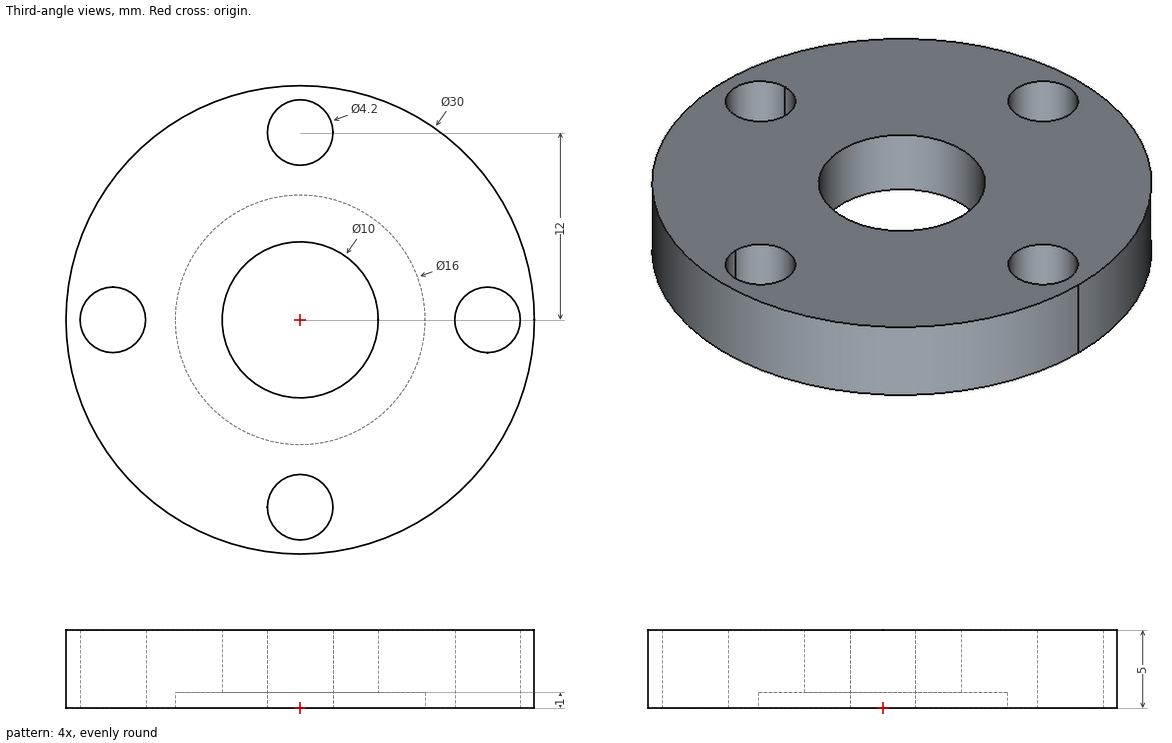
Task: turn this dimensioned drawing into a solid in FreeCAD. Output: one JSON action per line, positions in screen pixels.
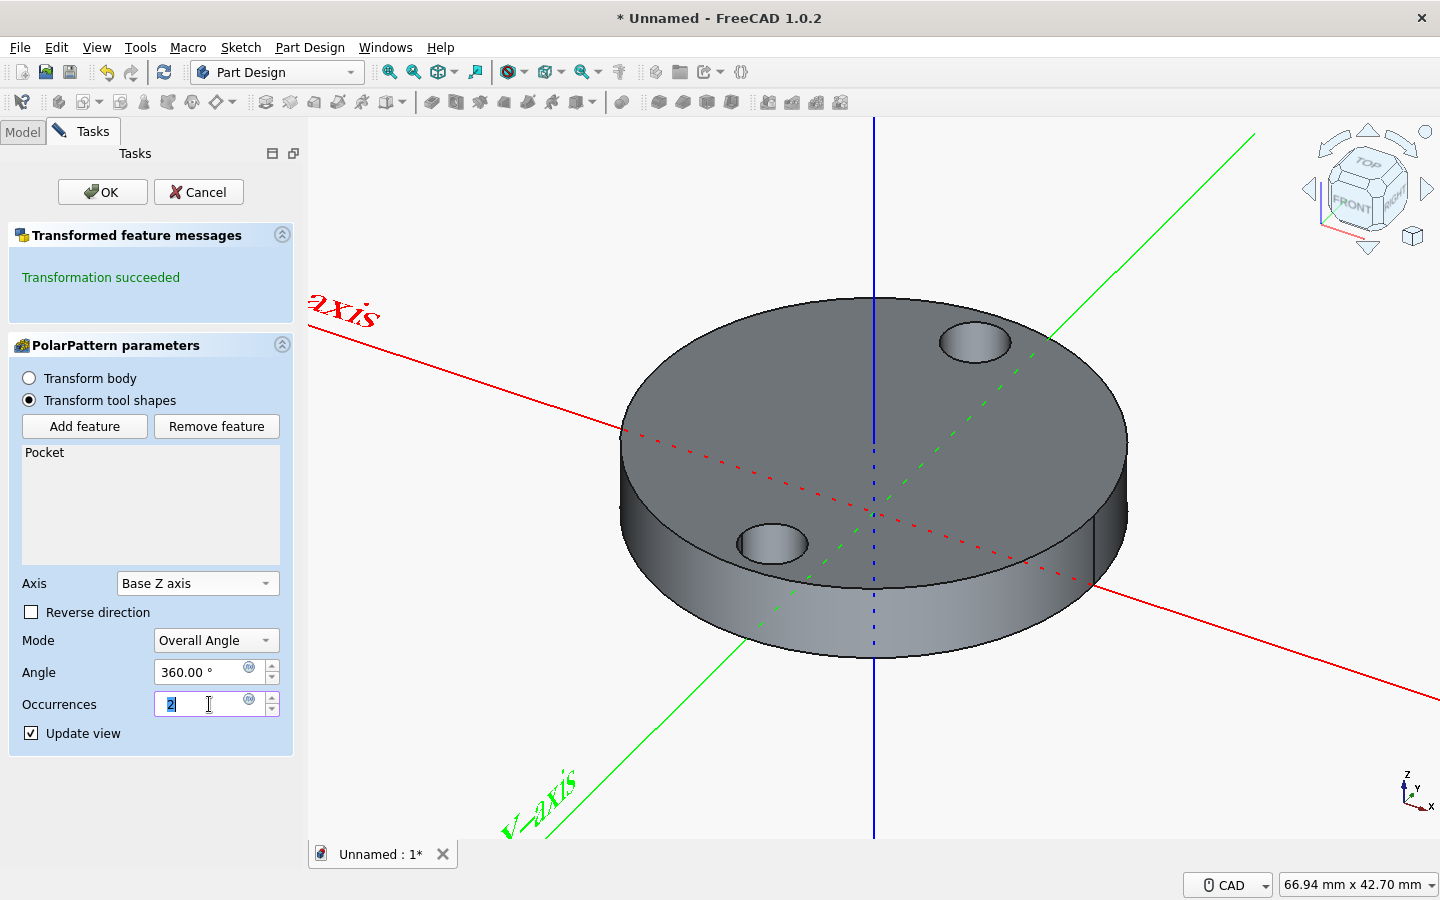
{"action": "type", "text": "4"}
{"action": "key", "text": "Tab"}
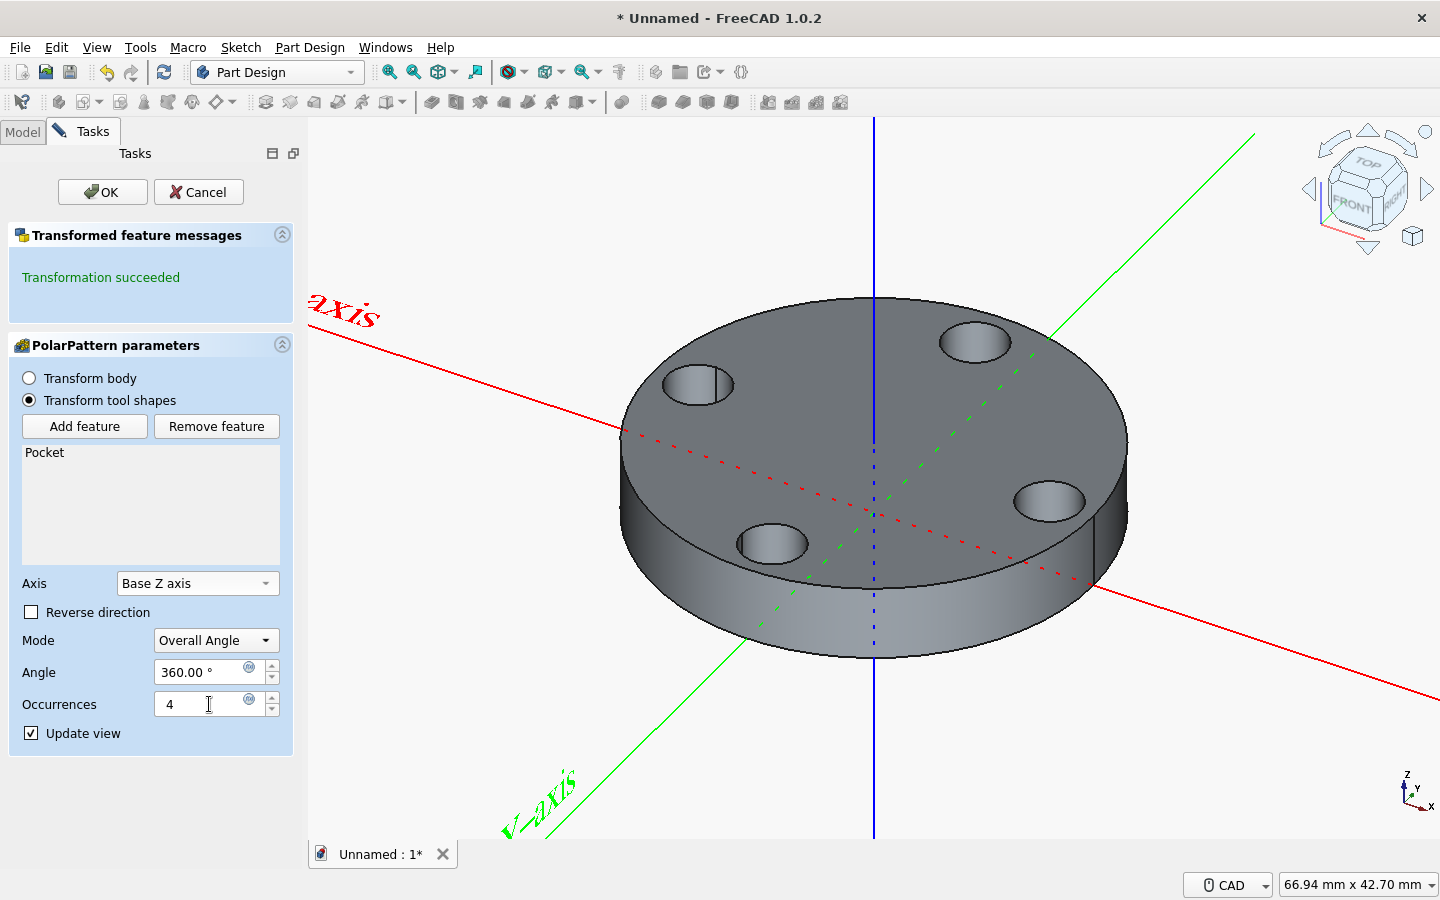
{"action": "left_click", "coordinate": [103, 192]}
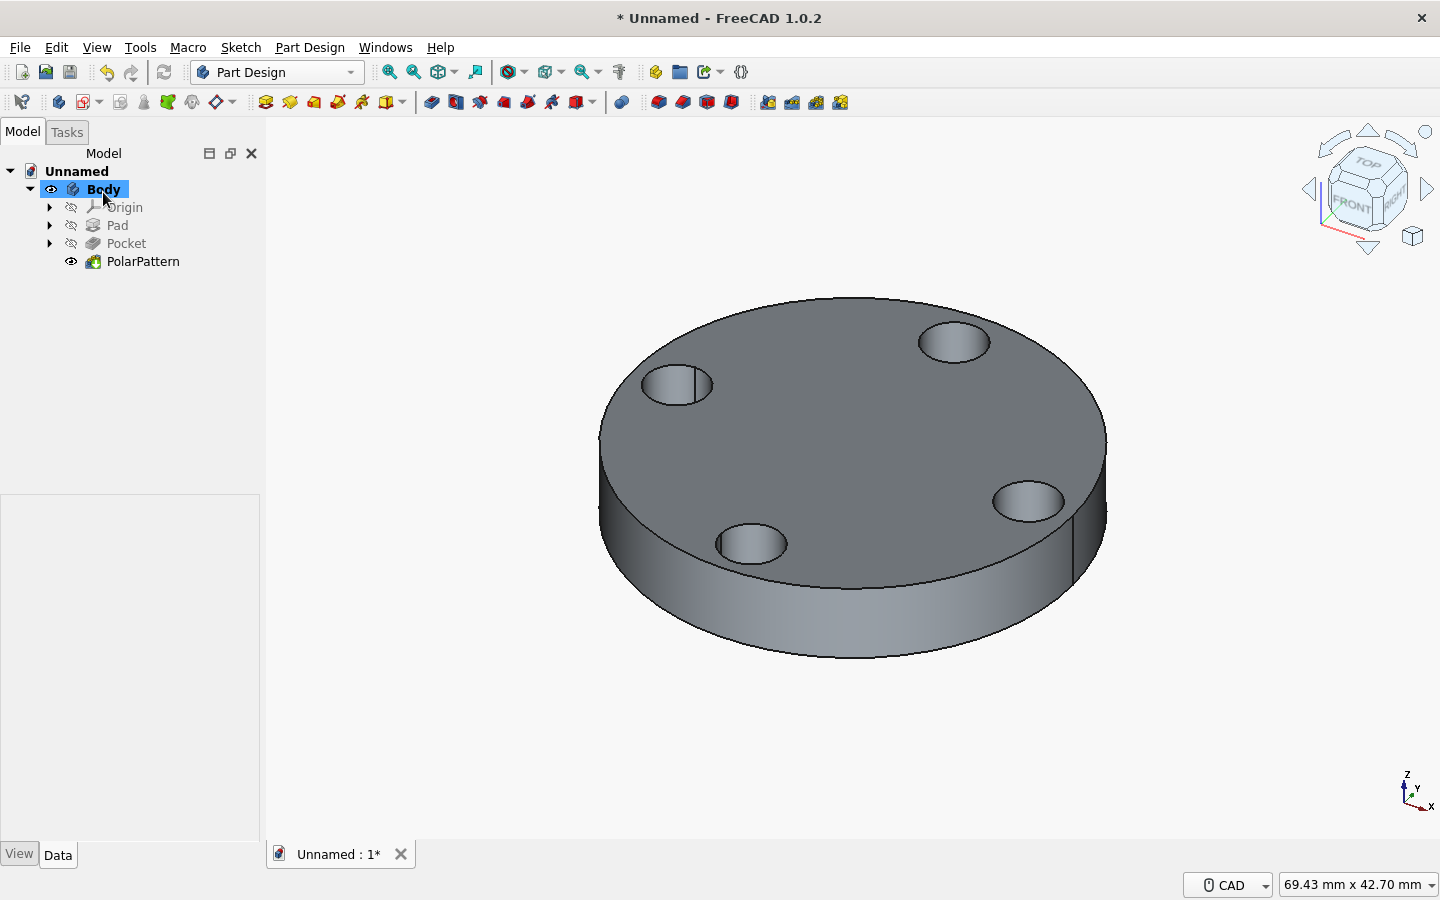
{"action": "key", "text": "5"}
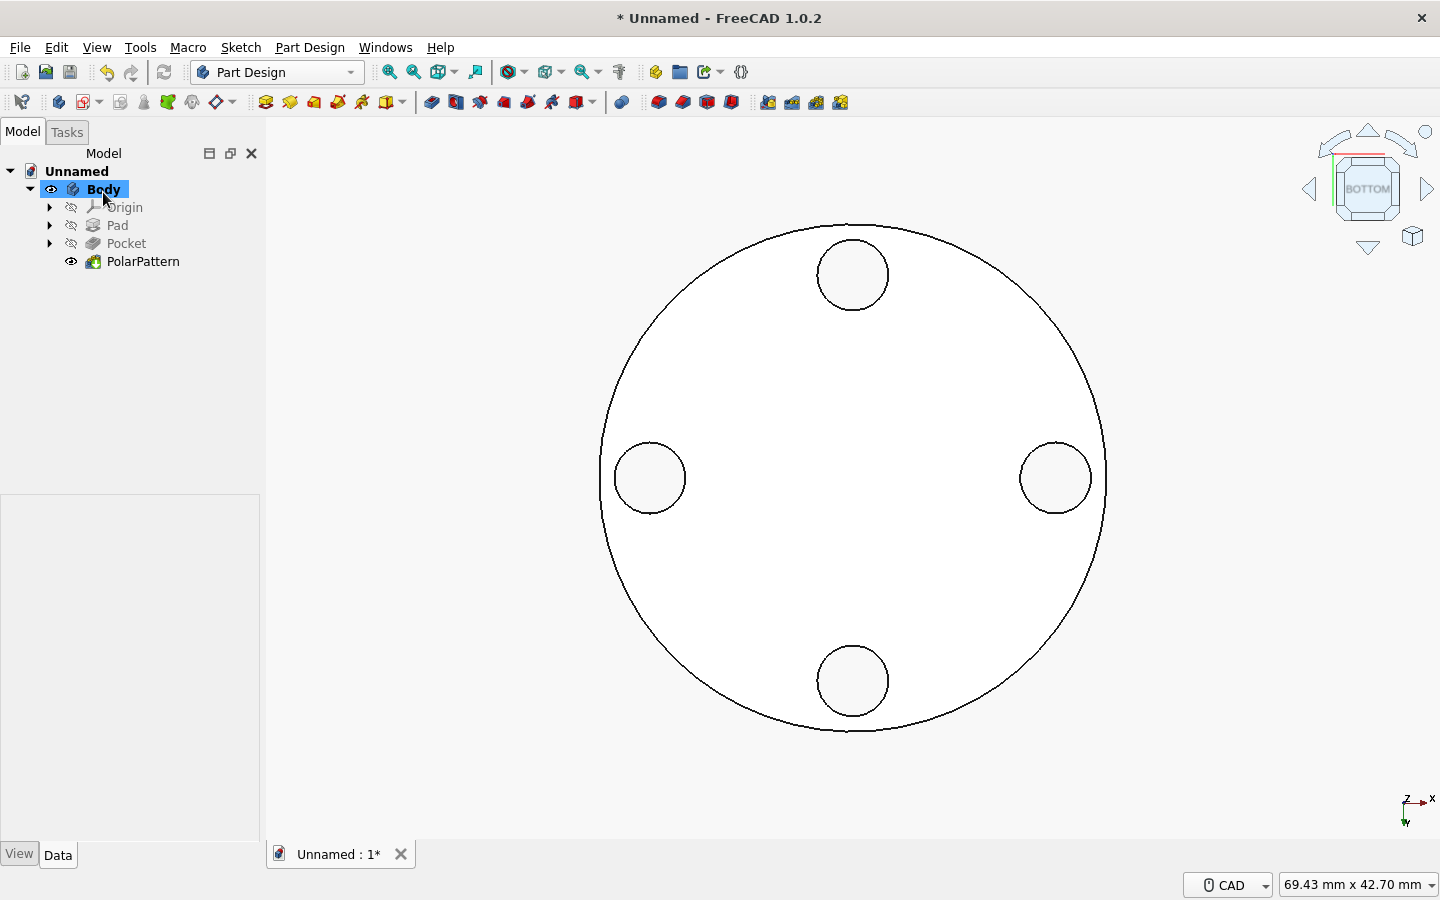
{"action": "left_click", "coordinate": [853, 477]}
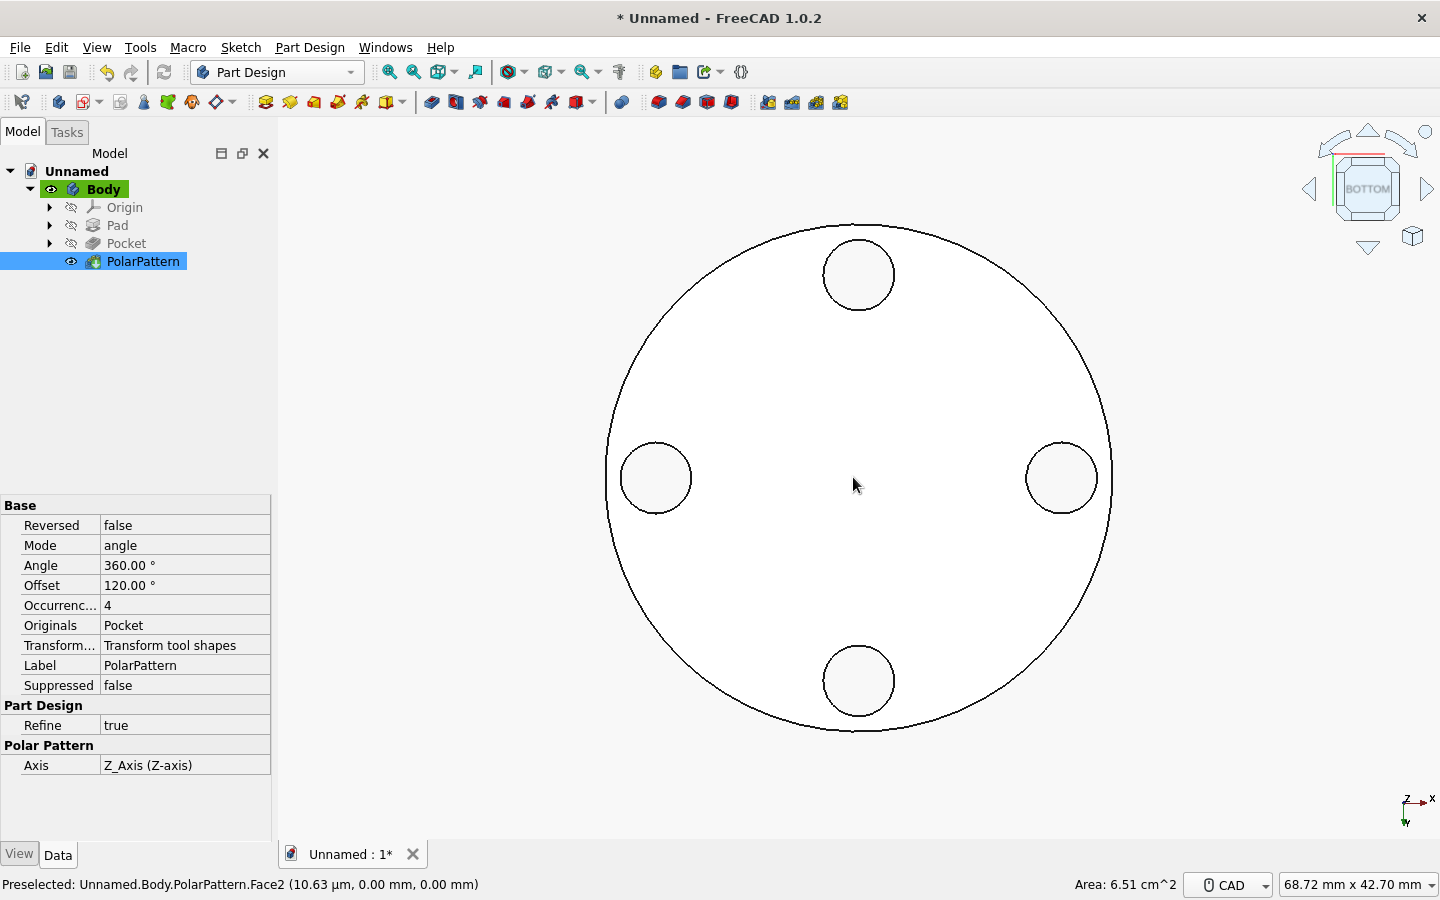
{"action": "left_click", "coordinate": [84, 102]}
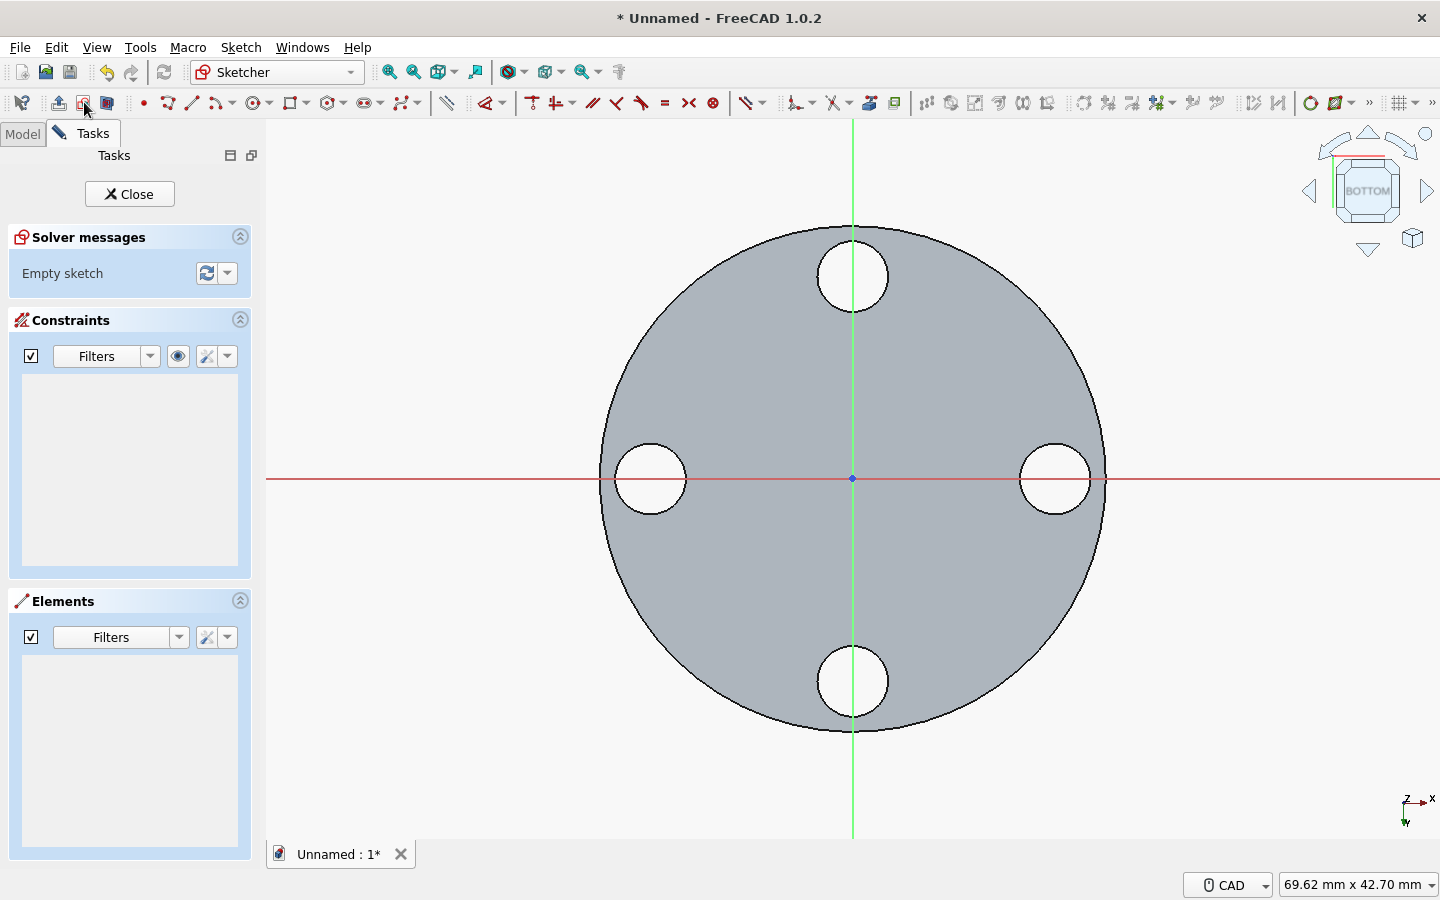
{"action": "scroll", "coordinate": [936, 479], "scroll_direction": "up", "scroll_amount": 3}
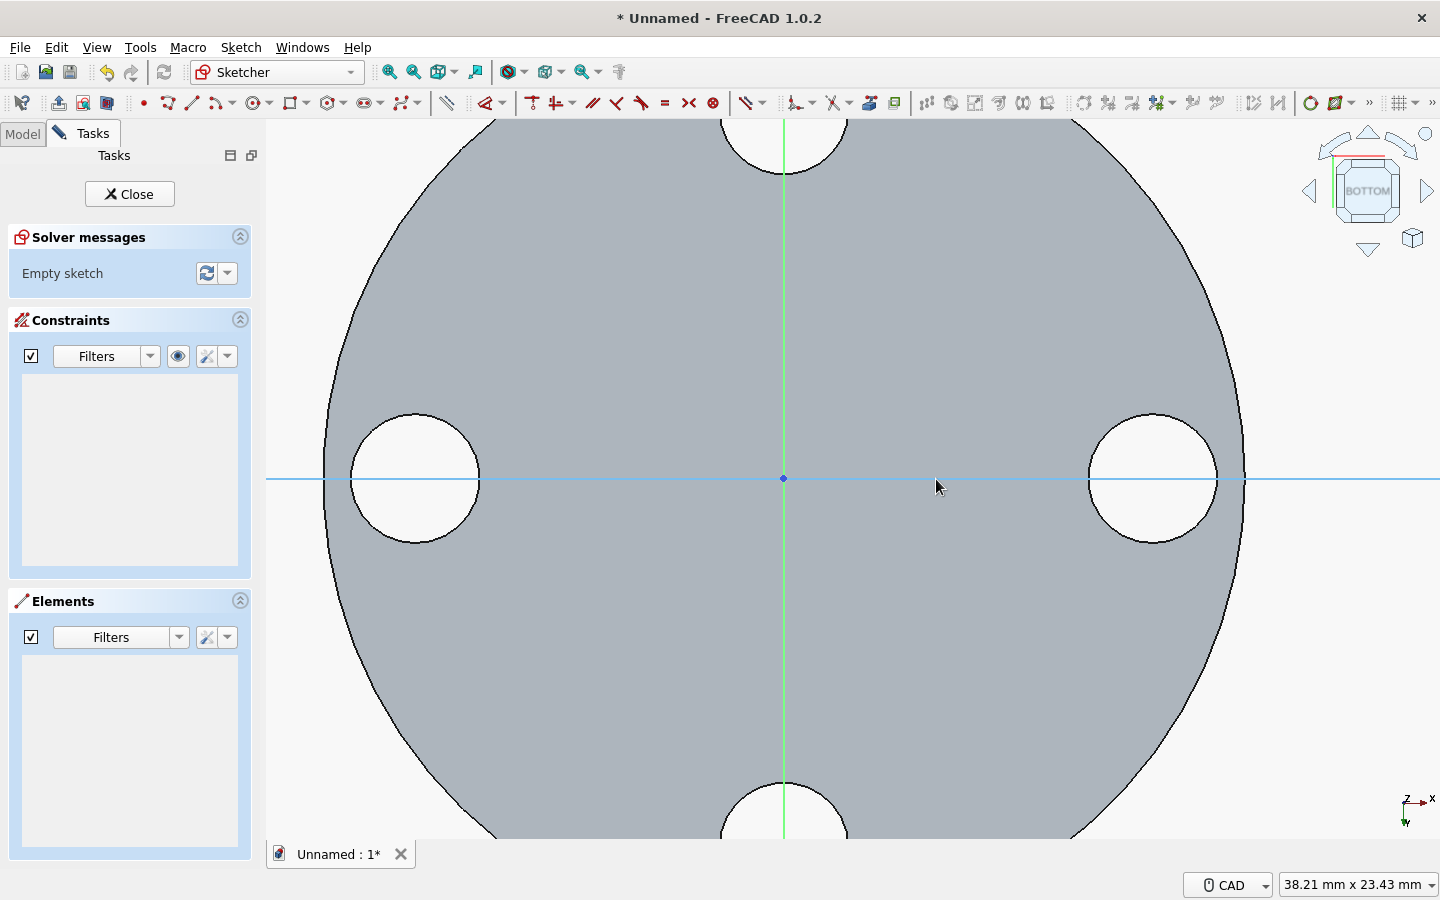
{"action": "left_click", "coordinate": [254, 104]}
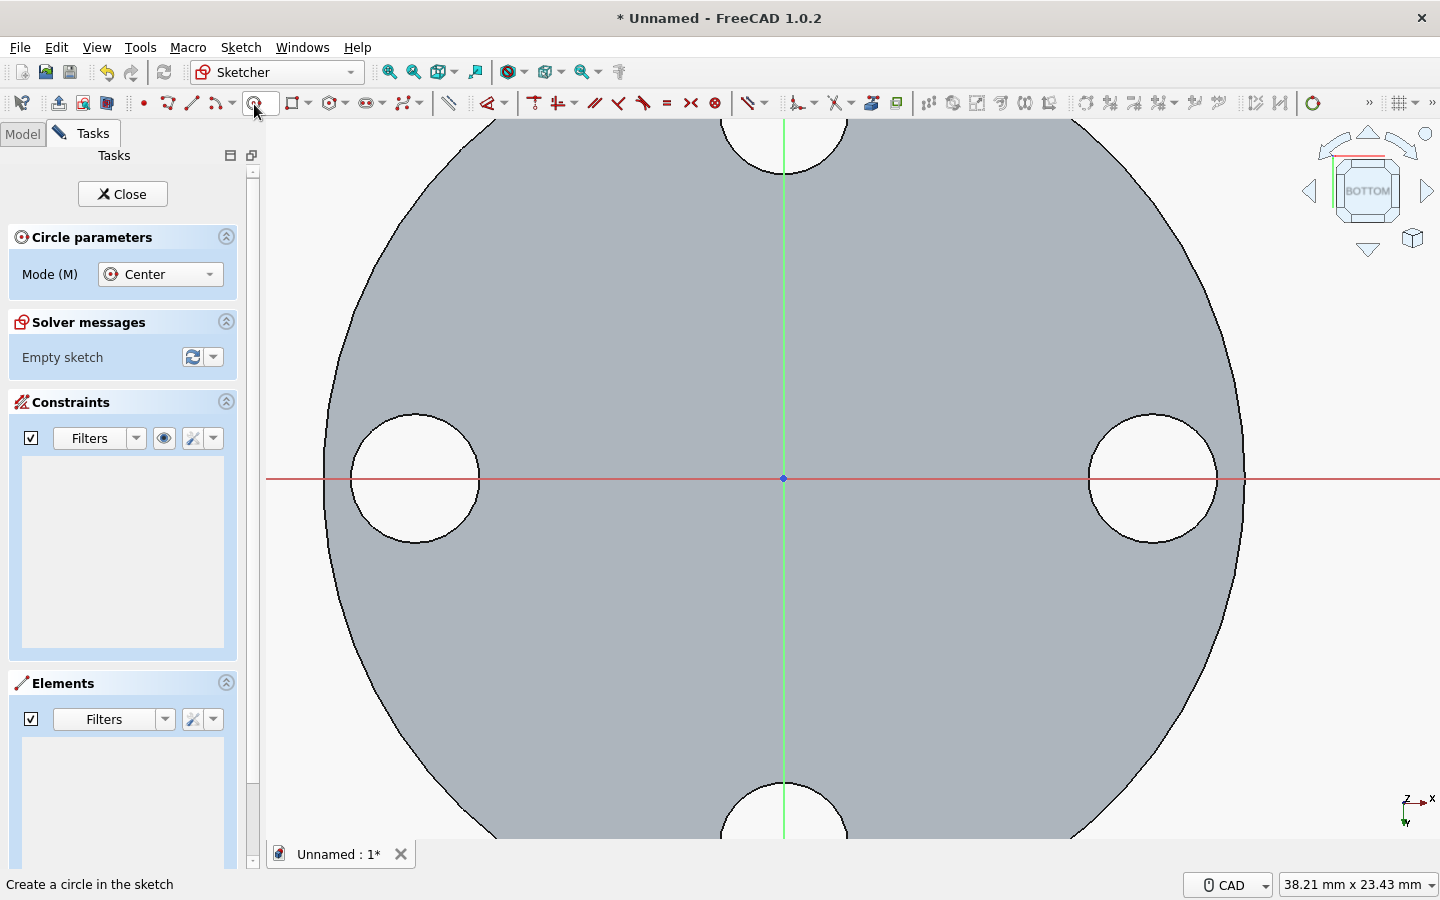
{"action": "left_click", "coordinate": [784, 479]}
{"action": "mouse_move", "coordinate": [958, 305]}